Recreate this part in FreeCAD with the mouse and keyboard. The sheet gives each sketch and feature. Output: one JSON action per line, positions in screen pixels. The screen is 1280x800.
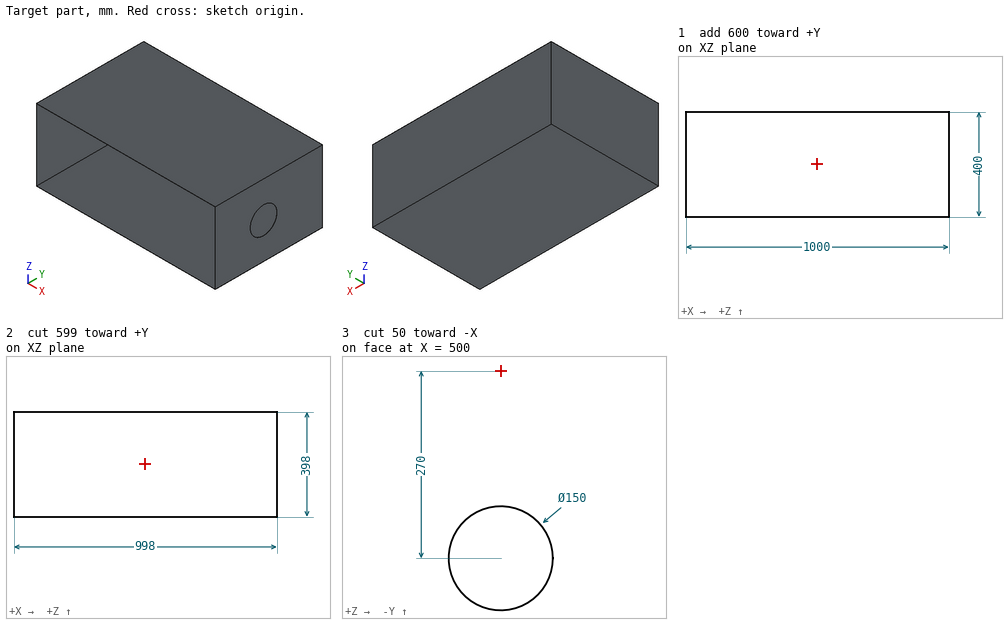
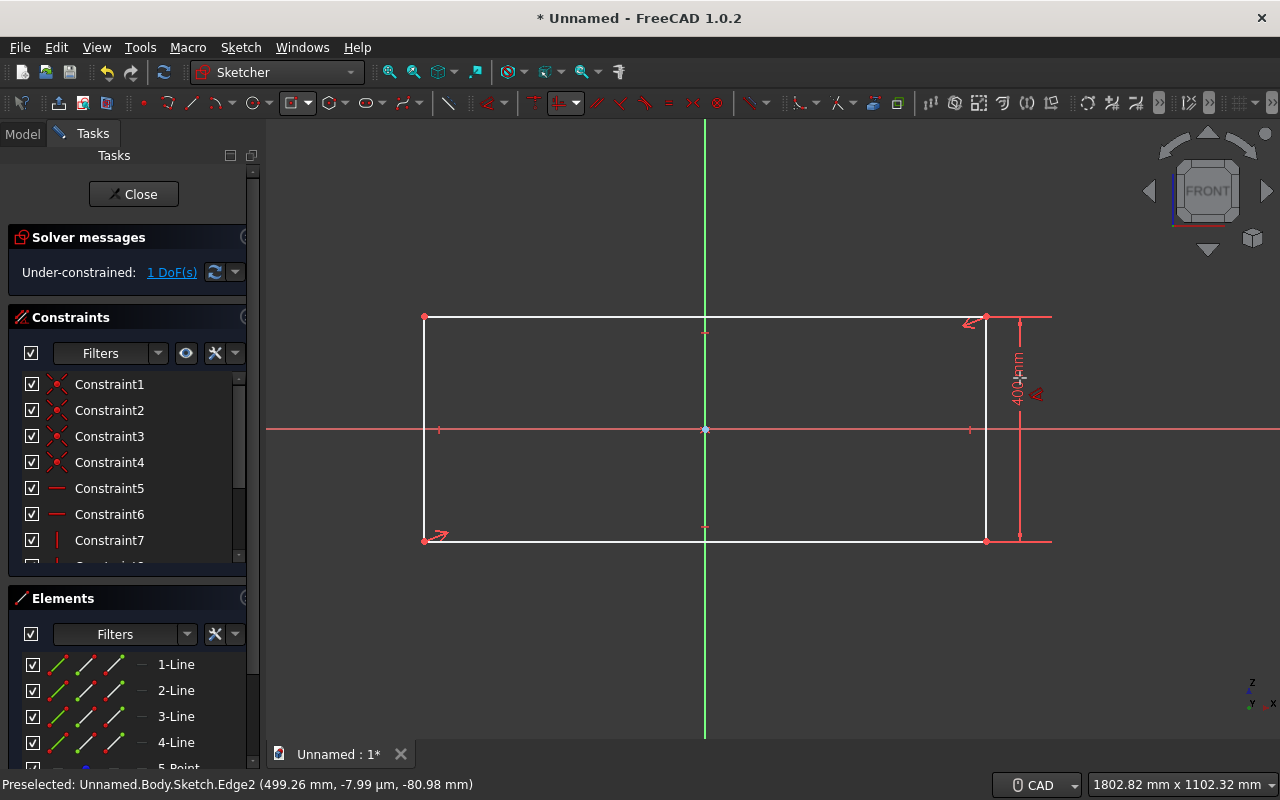
{"action": "left_click", "coordinate": [593, 542]}
{"action": "left_click", "coordinate": [576, 576]}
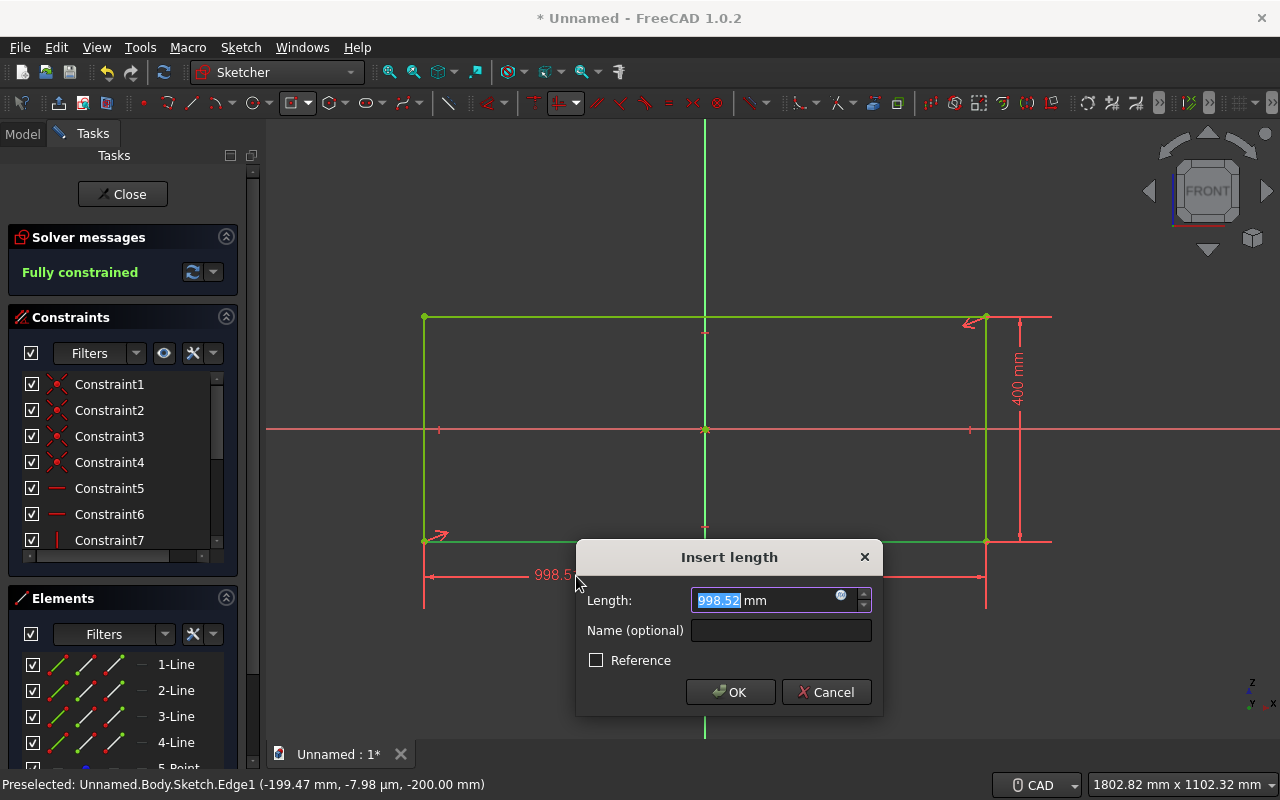
{"action": "type", "text": "1000"}
{"action": "key", "text": "Return"}
{"action": "key", "text": "Escape"}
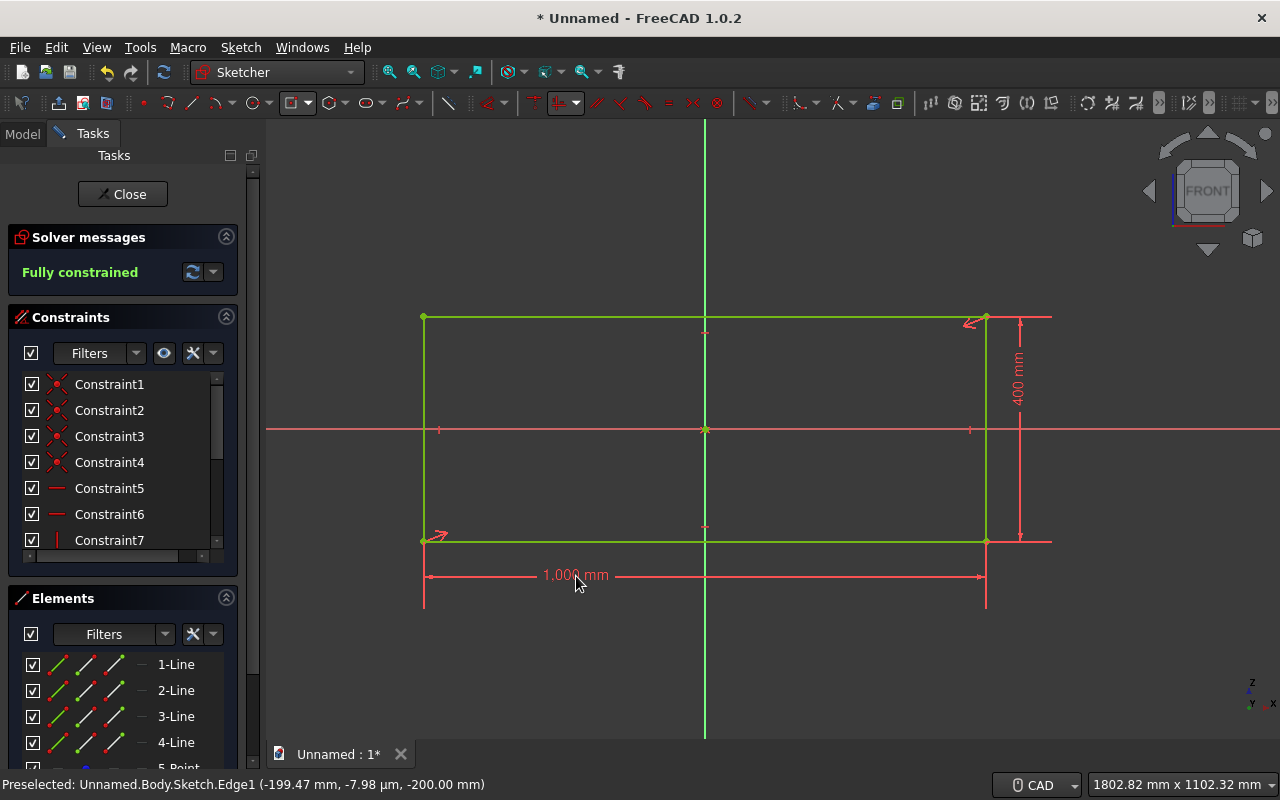
{"action": "left_click", "coordinate": [123, 194]}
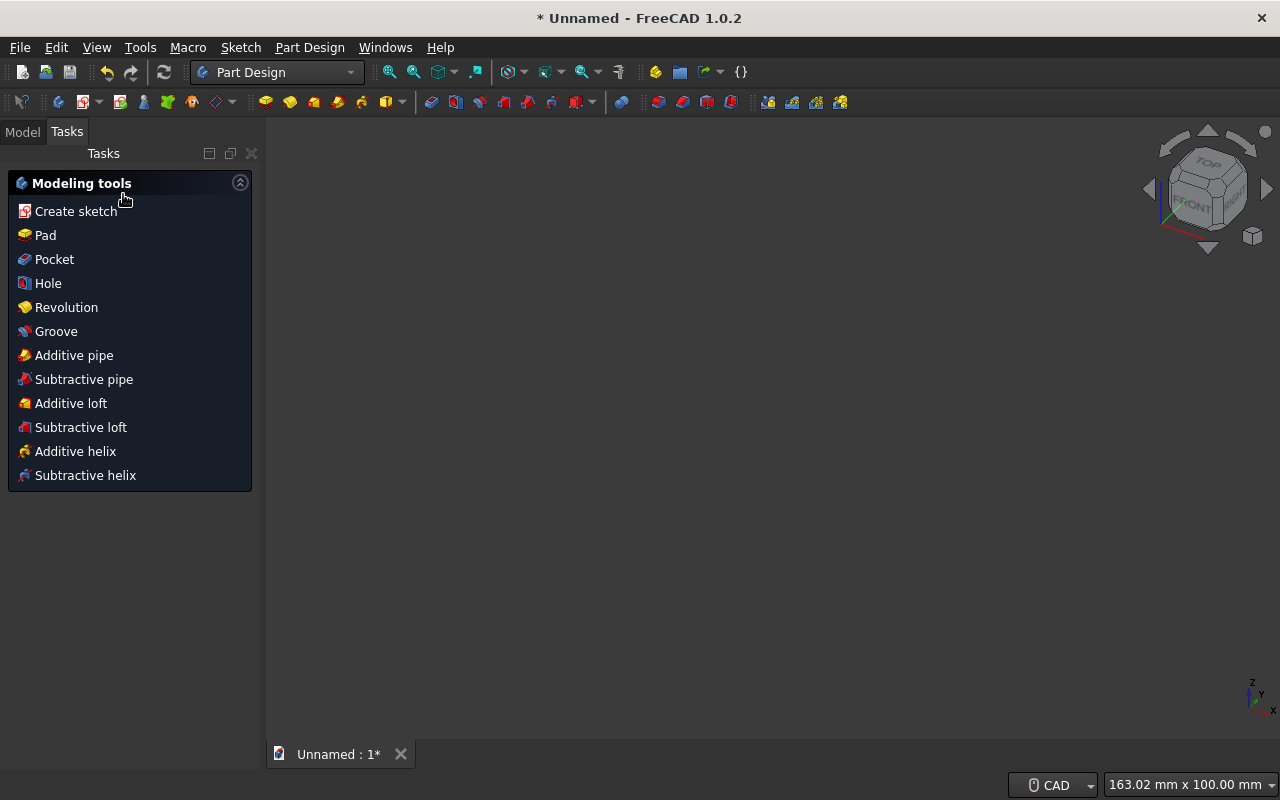
{"action": "left_click", "coordinate": [266, 102]}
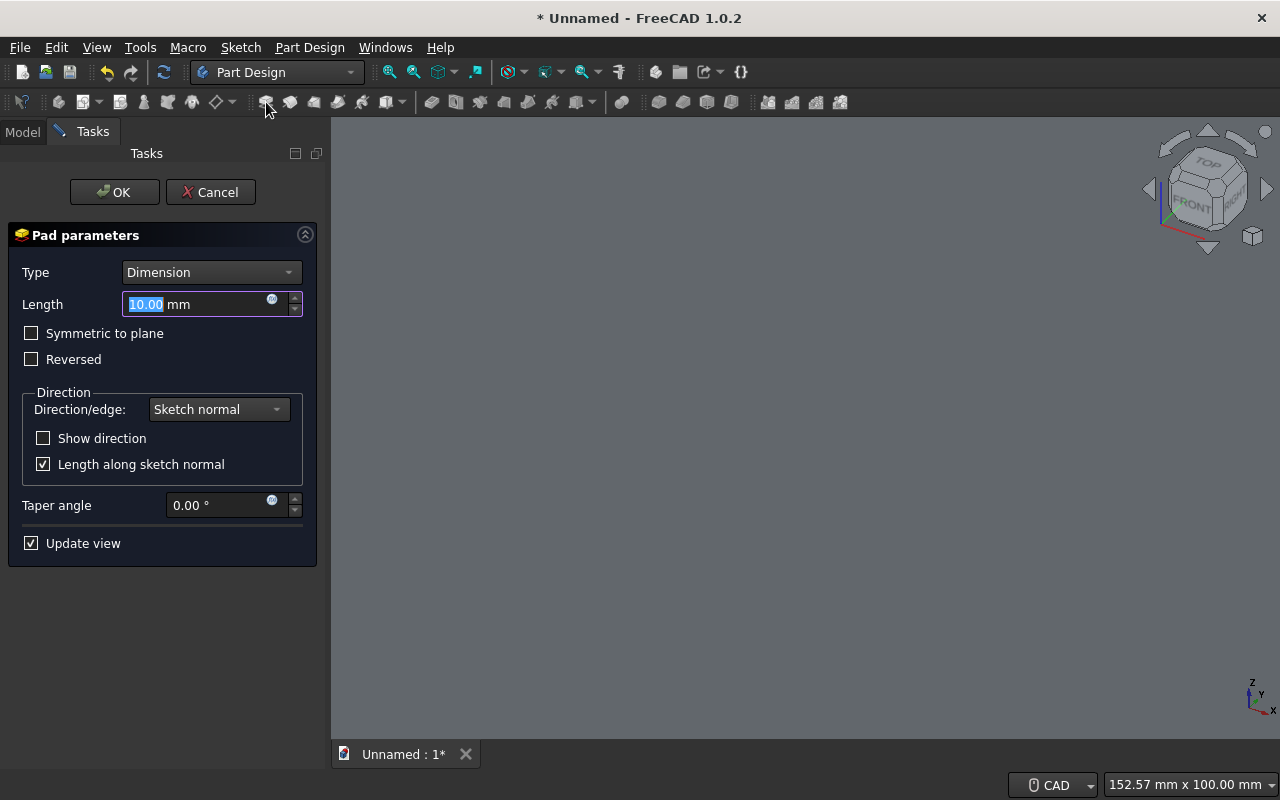
{"action": "type", "text": "600"}
{"action": "key", "text": "Tab"}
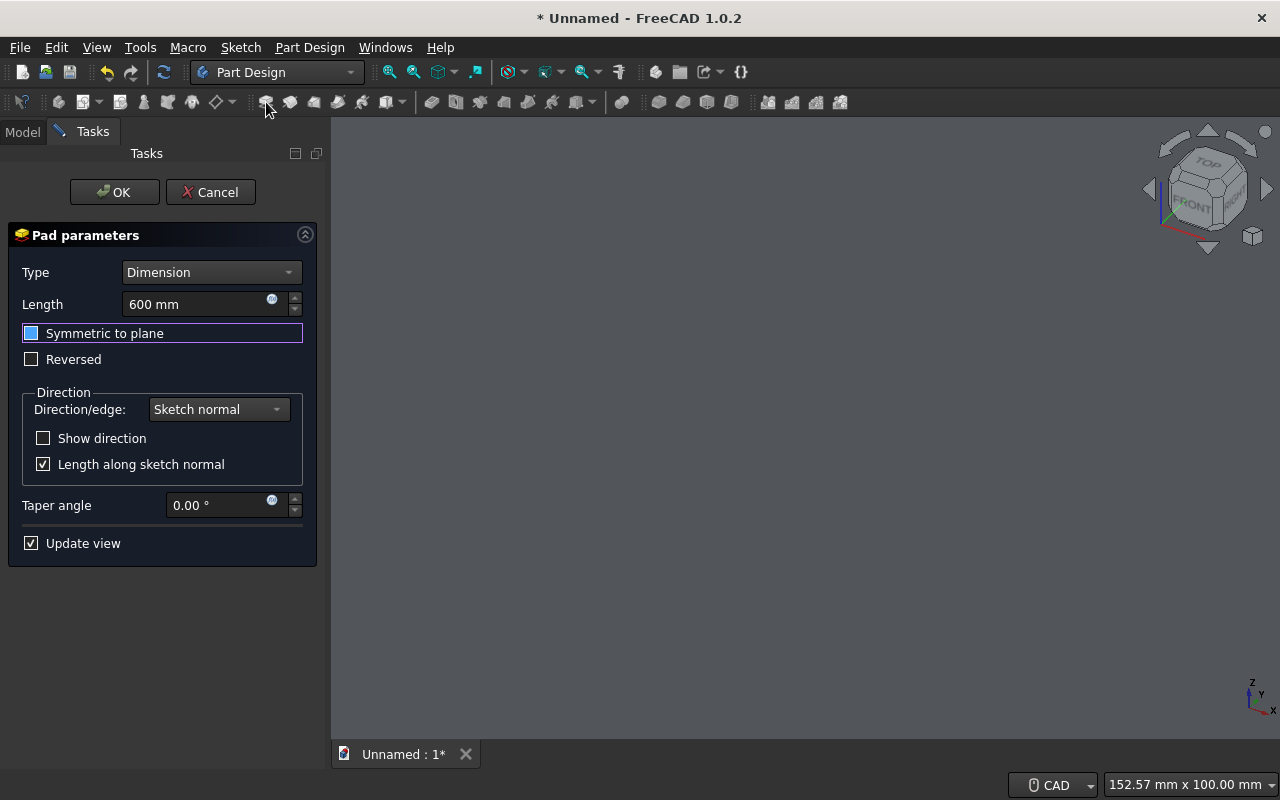
{"action": "left_click", "coordinate": [30, 359]}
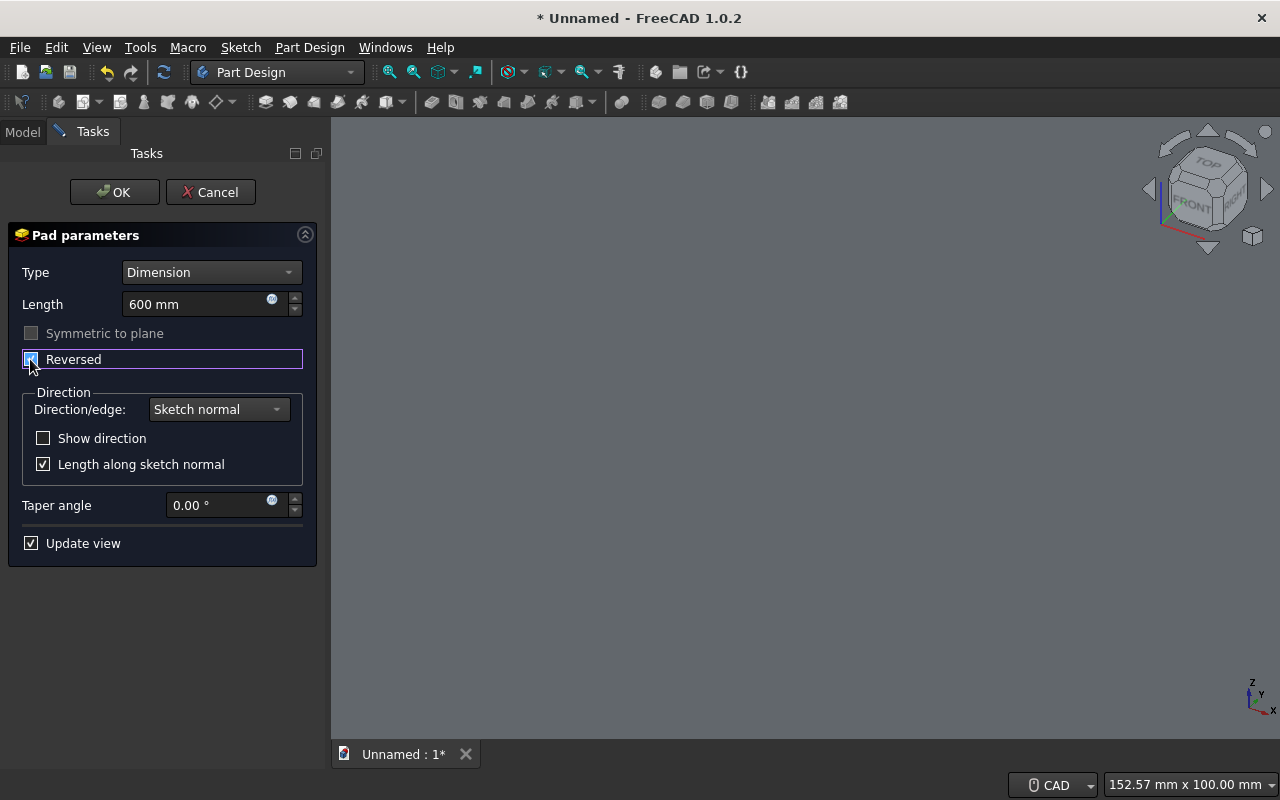
{"action": "left_click", "coordinate": [115, 192]}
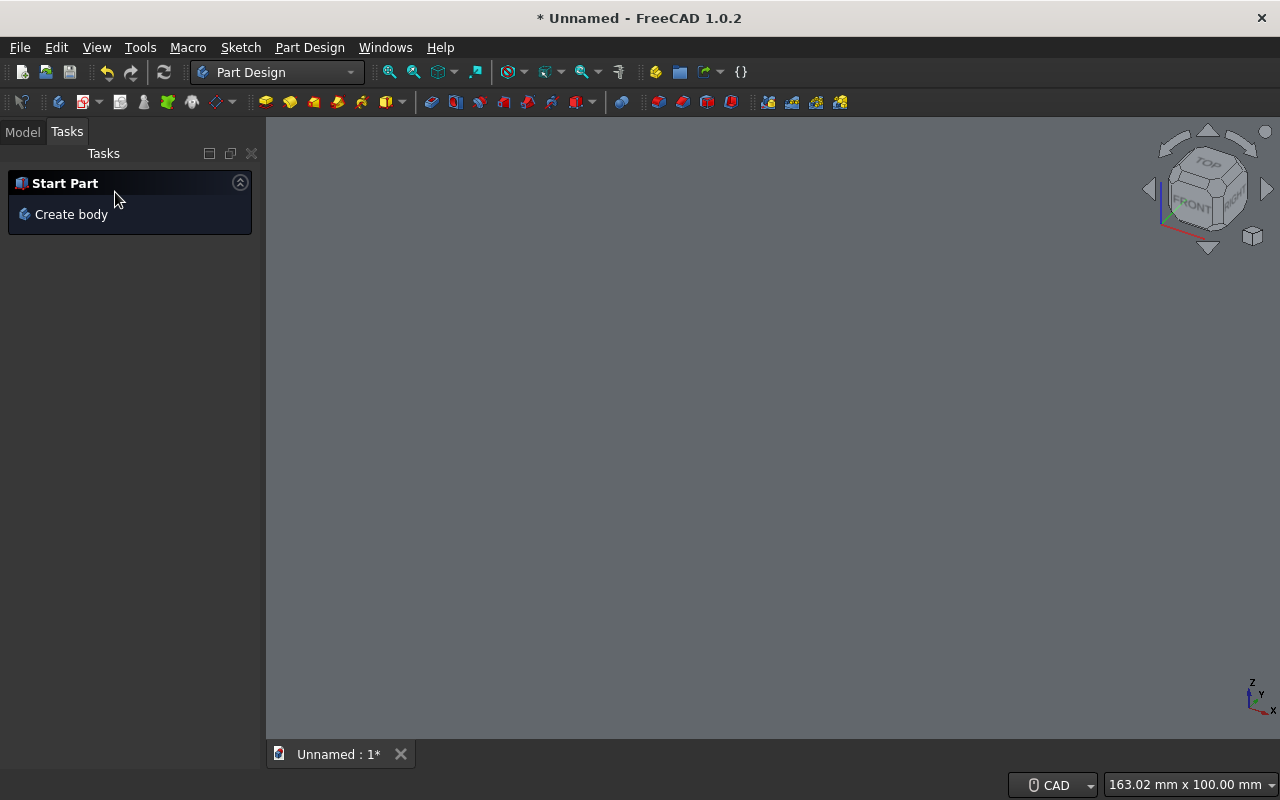
{"action": "key", "text": "v f"}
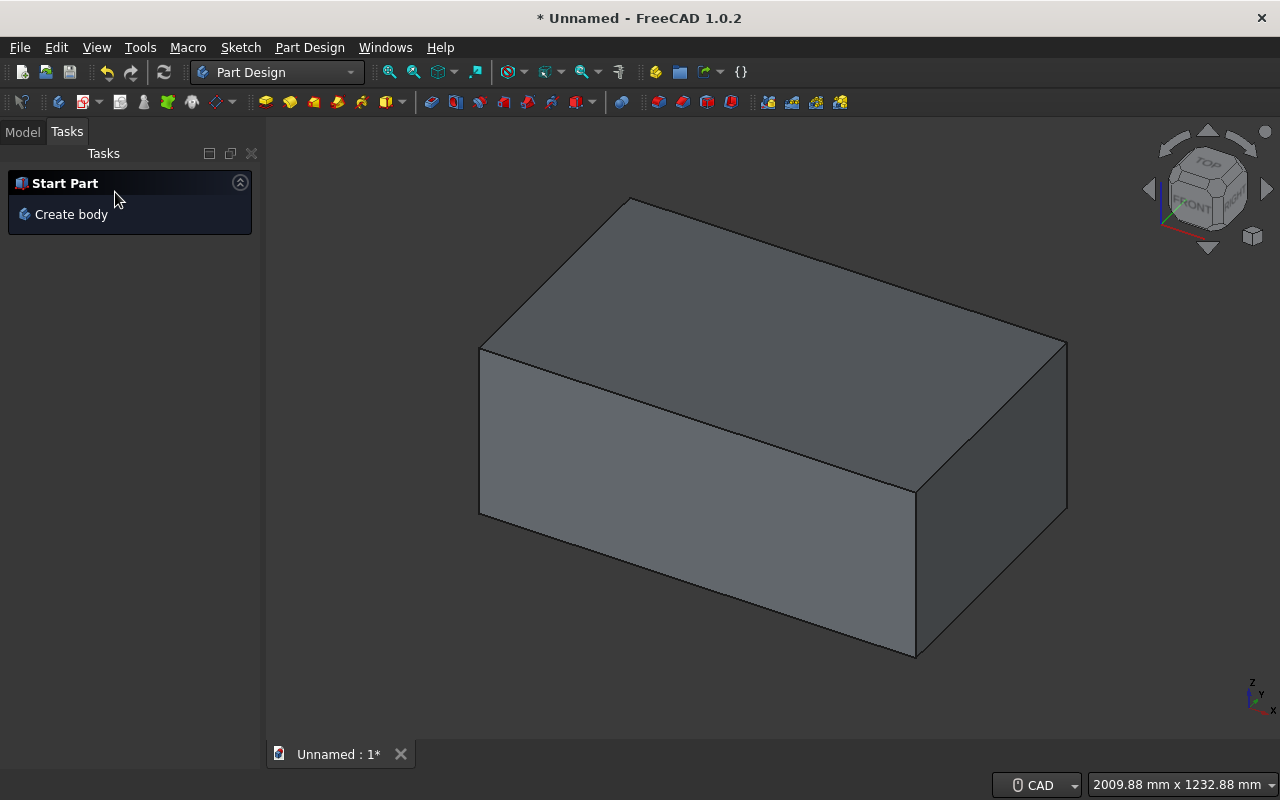
{"action": "left_click", "coordinate": [84, 102]}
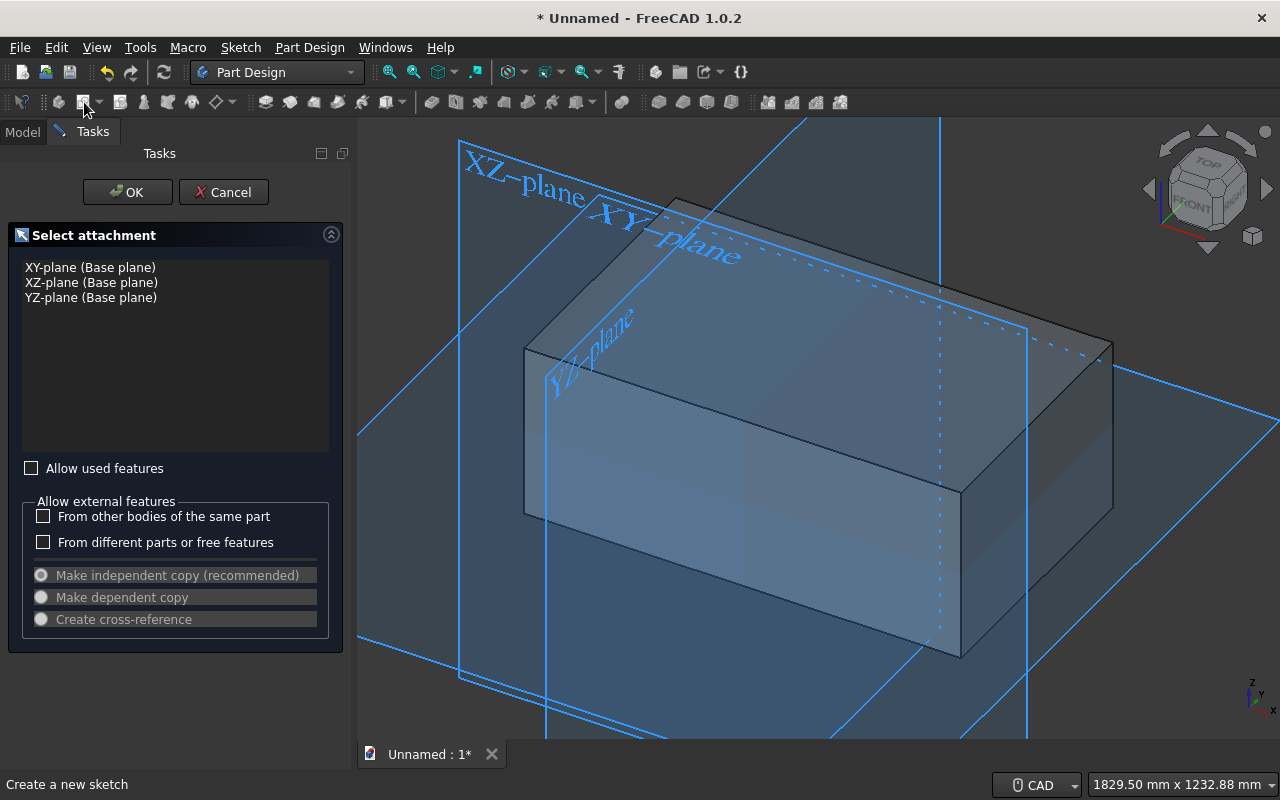
{"action": "left_click", "coordinate": [82, 282]}